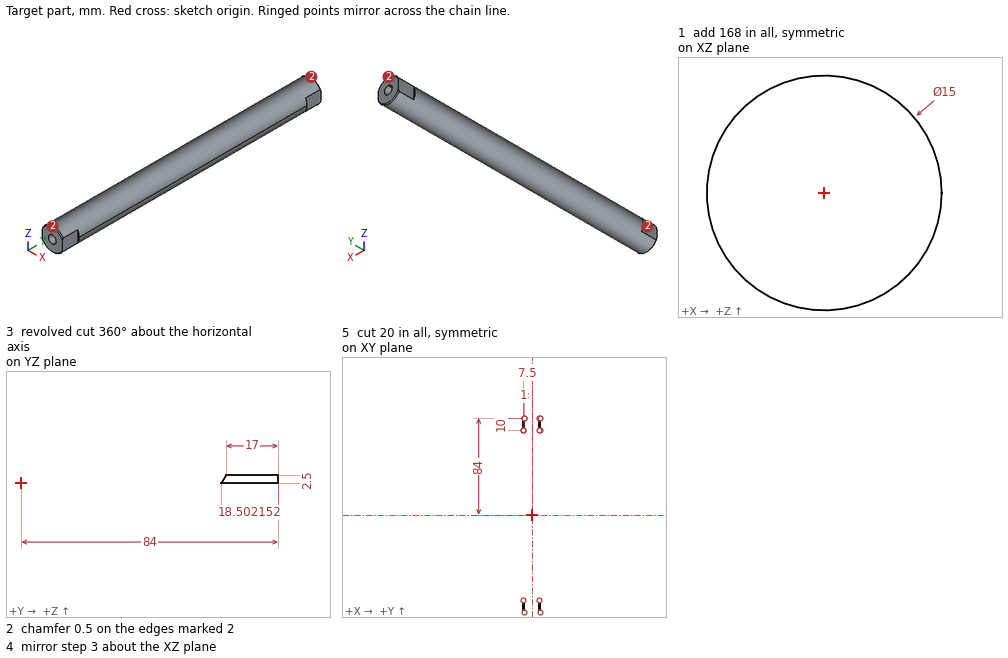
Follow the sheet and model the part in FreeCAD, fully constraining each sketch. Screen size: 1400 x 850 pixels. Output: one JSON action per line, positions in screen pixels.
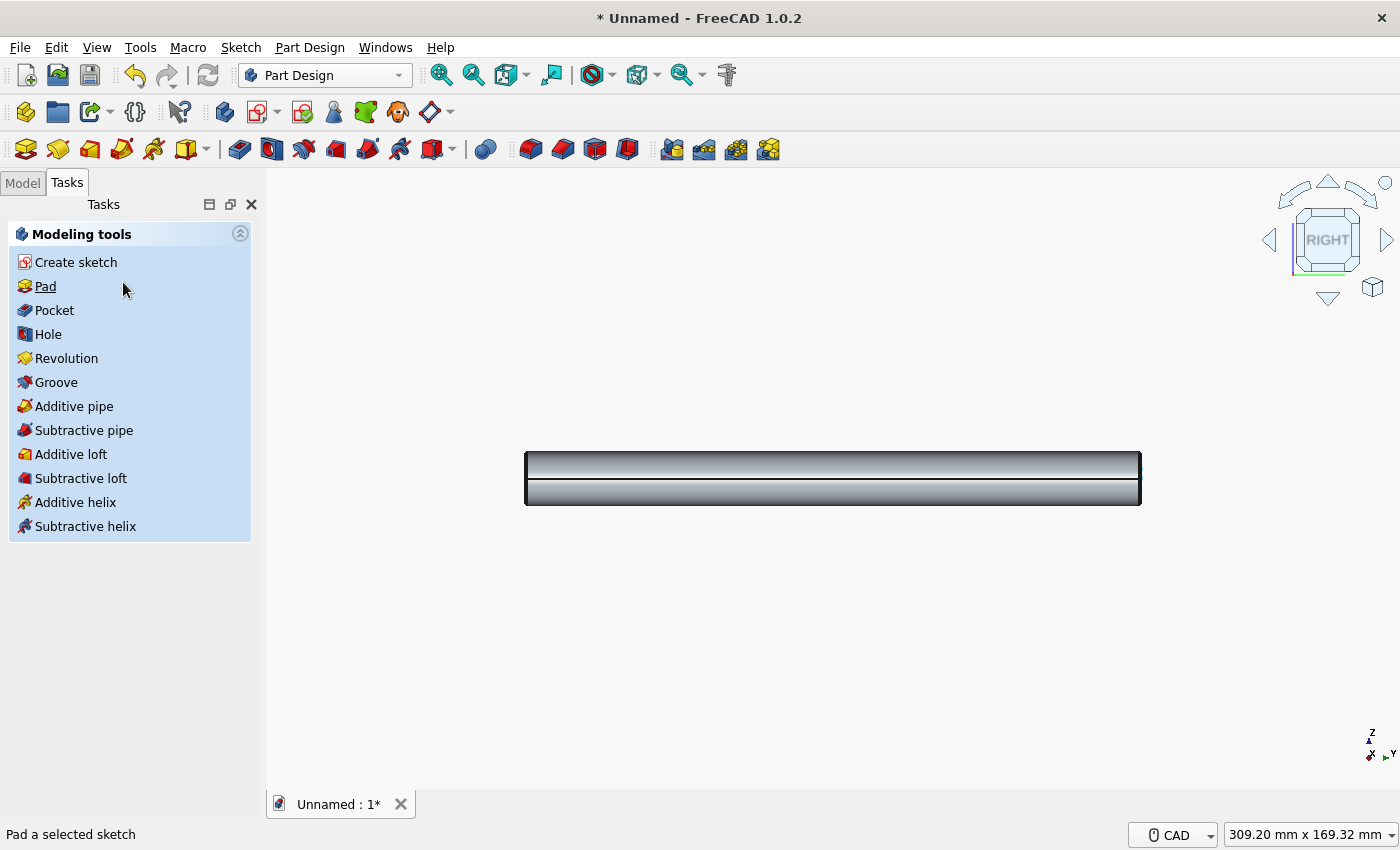
{"action": "left_click", "coordinate": [304, 150]}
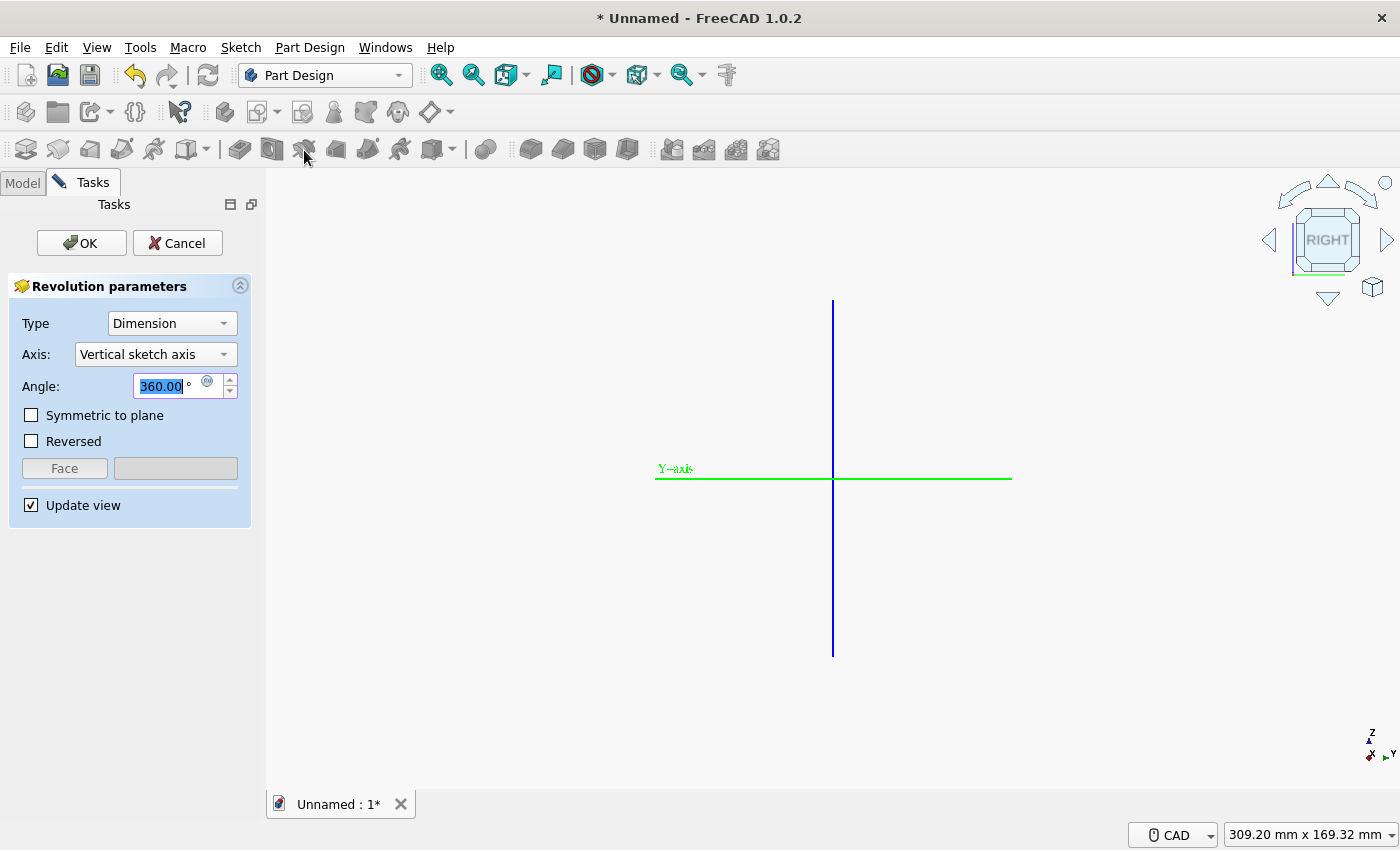
{"action": "left_click", "coordinate": [156, 354]}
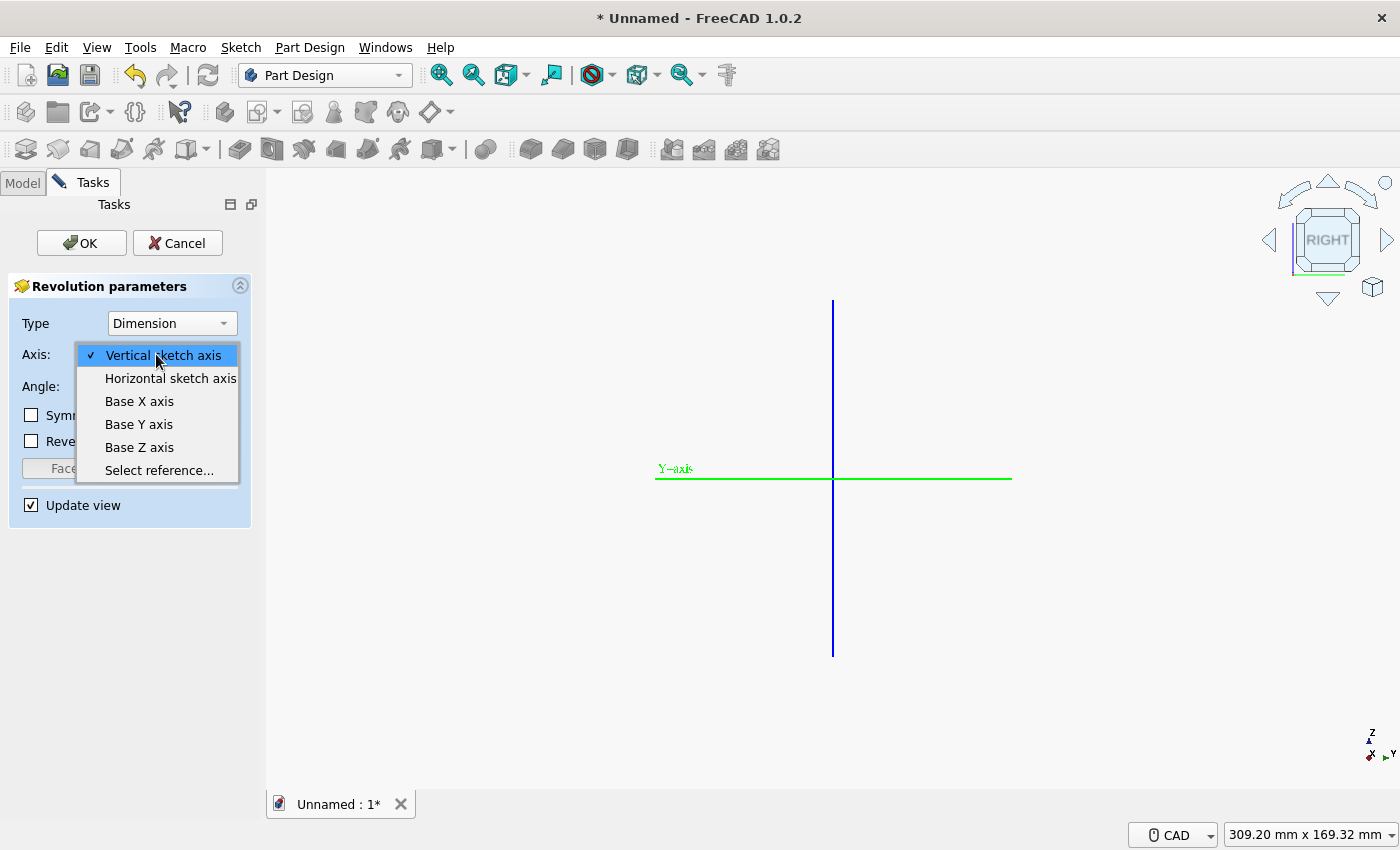
{"action": "left_click", "coordinate": [156, 378]}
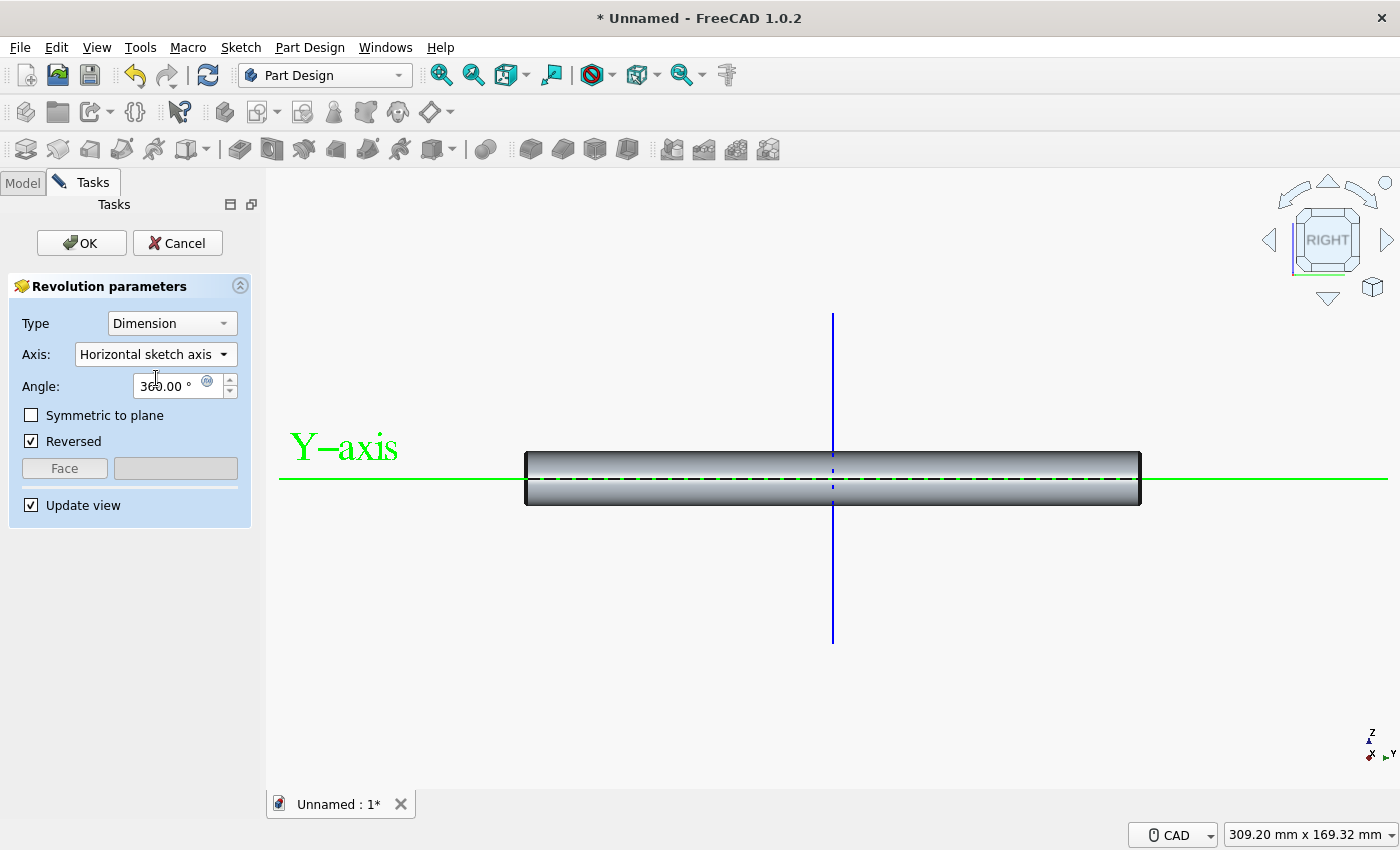
{"action": "left_click", "coordinate": [82, 243]}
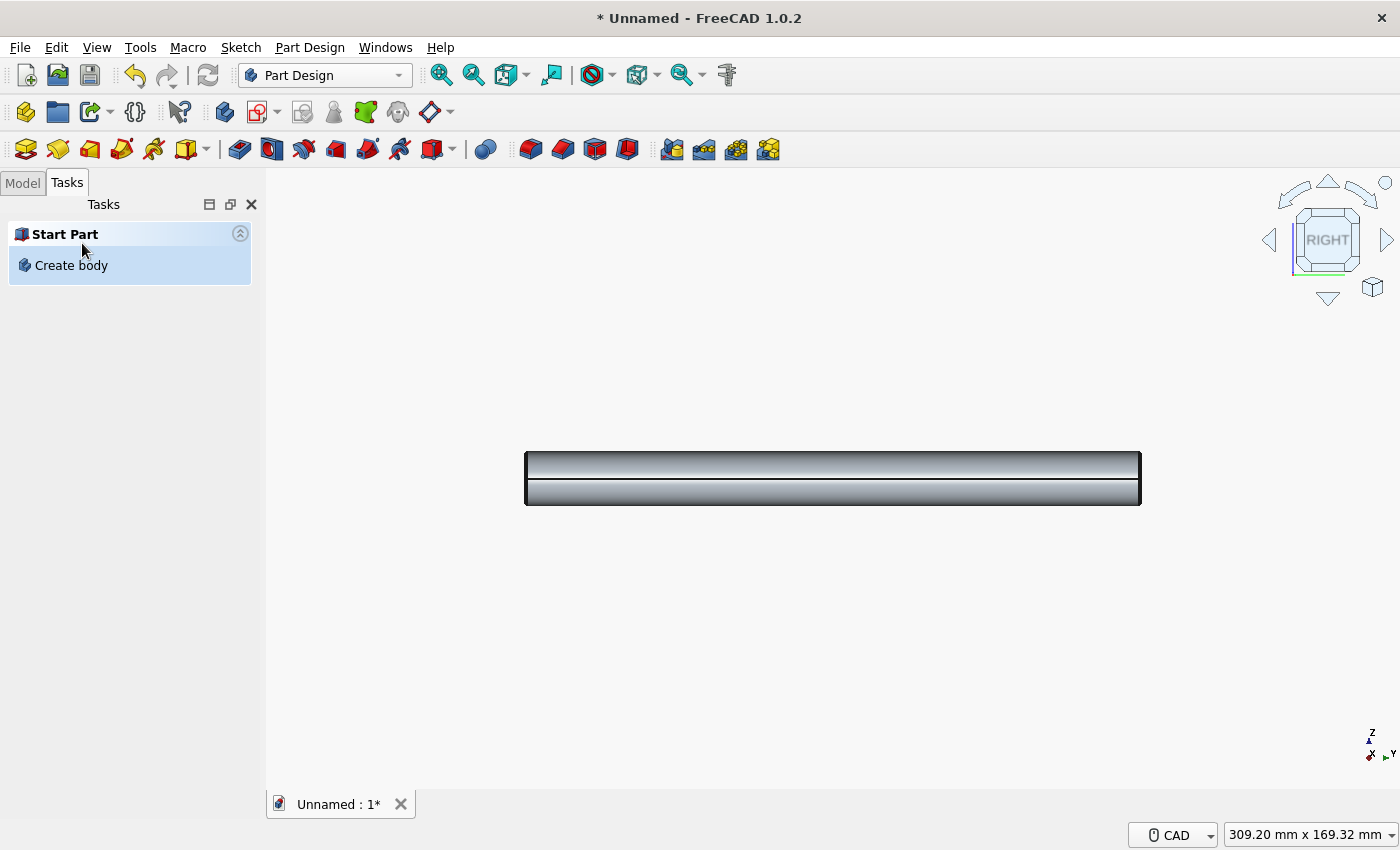
{"action": "left_click", "coordinate": [23, 182]}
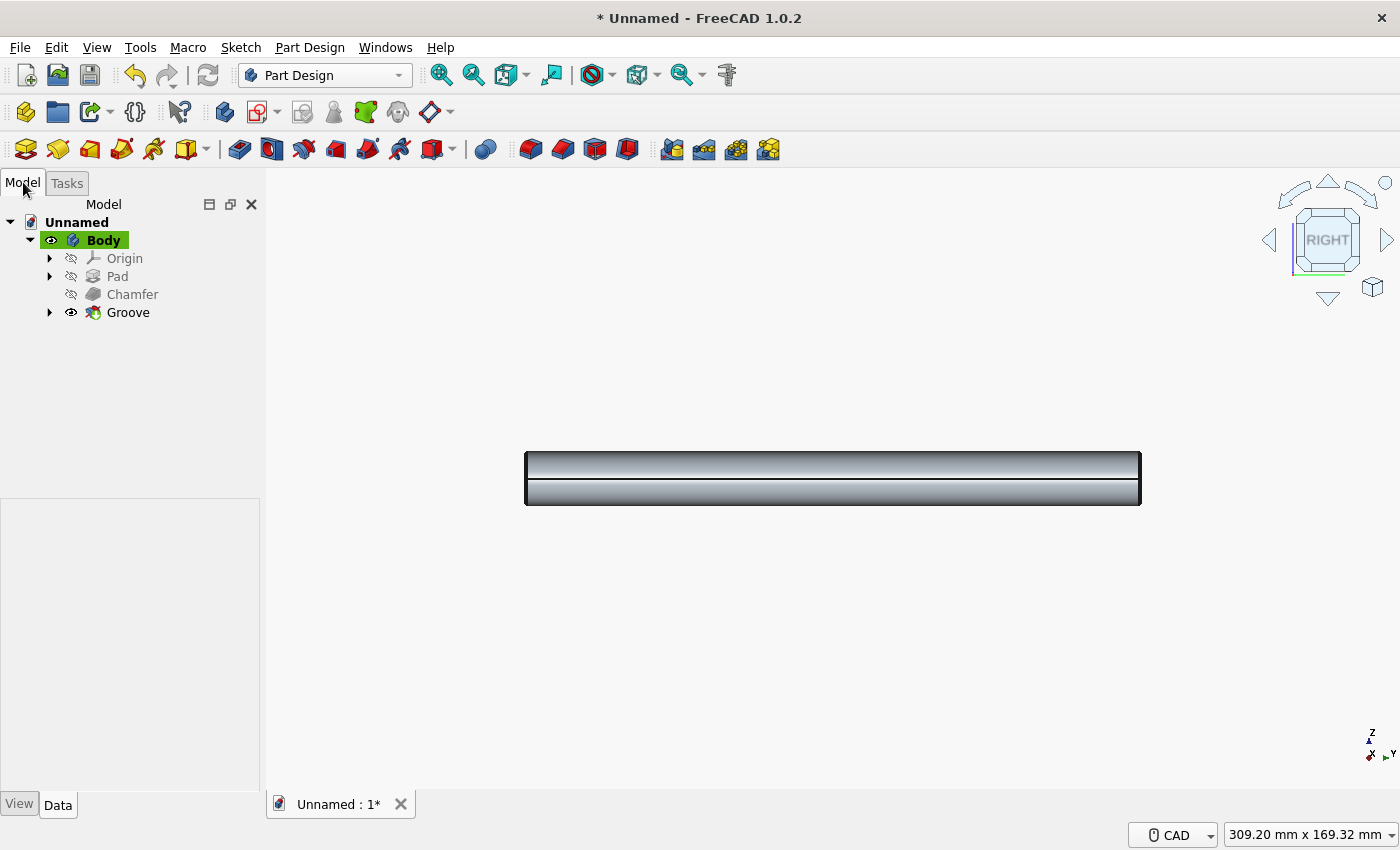
{"action": "left_click", "coordinate": [116, 312]}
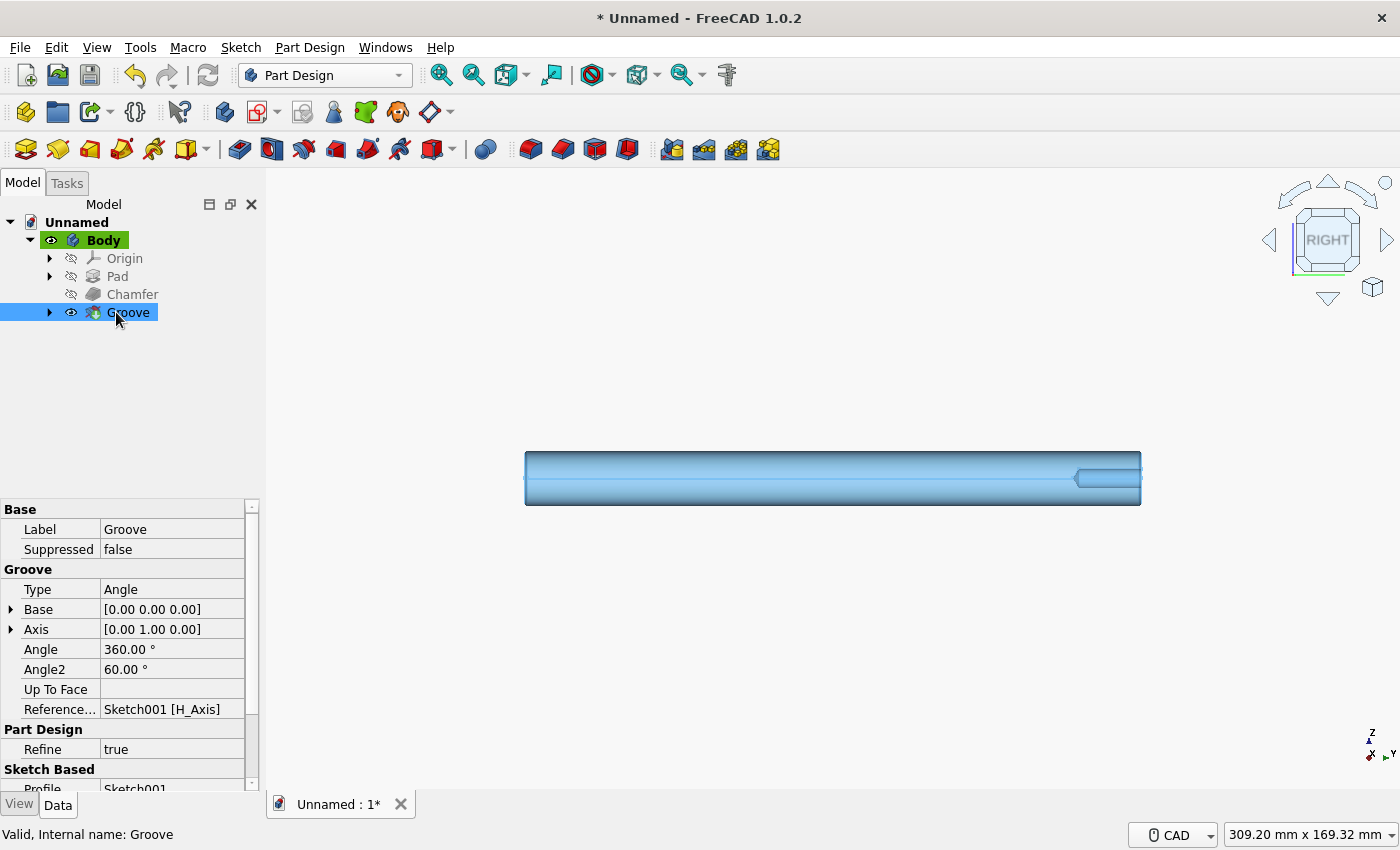
{"action": "left_click", "coordinate": [672, 150]}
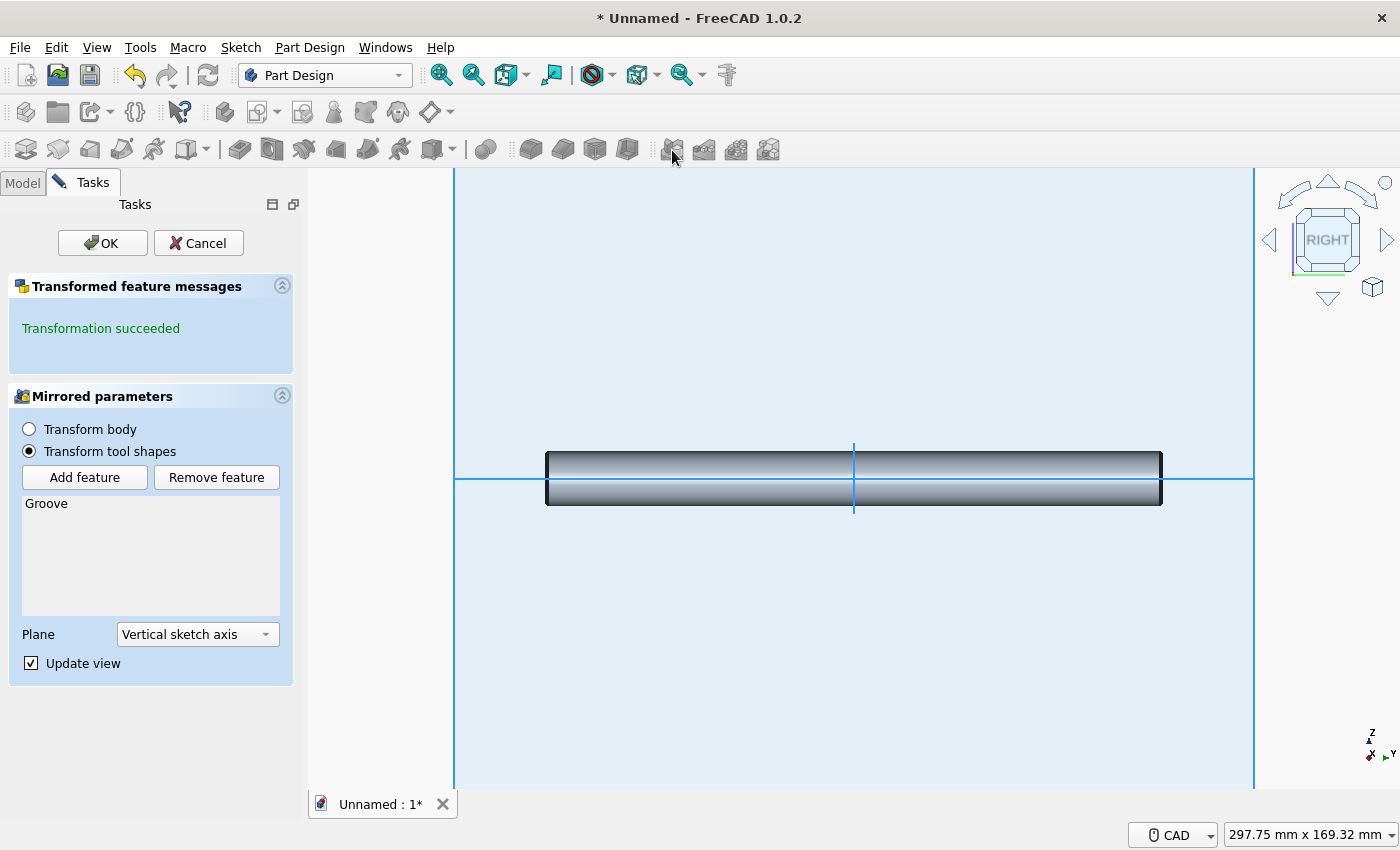
{"action": "left_click", "coordinate": [198, 634]}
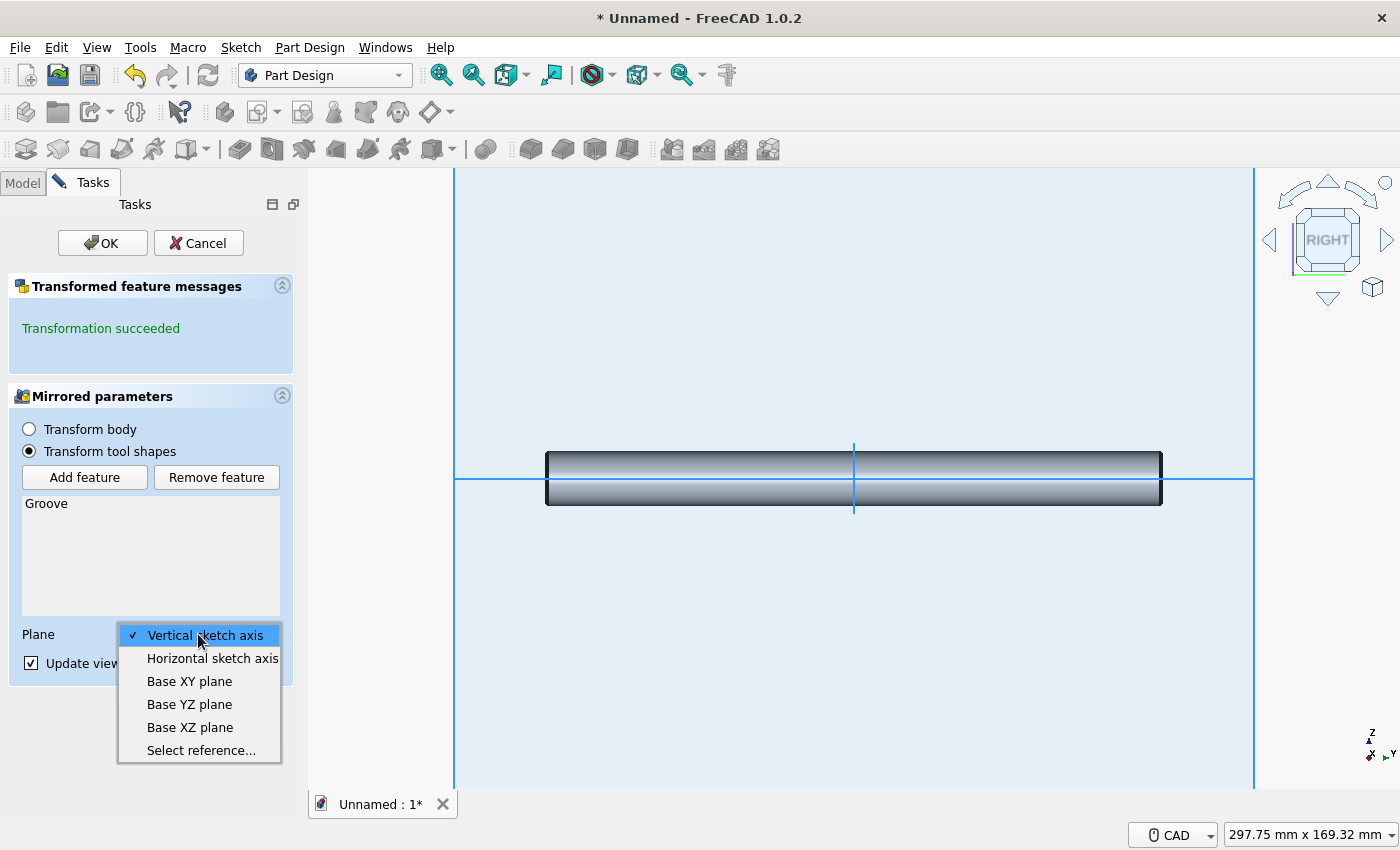
{"action": "left_click", "coordinate": [198, 728]}